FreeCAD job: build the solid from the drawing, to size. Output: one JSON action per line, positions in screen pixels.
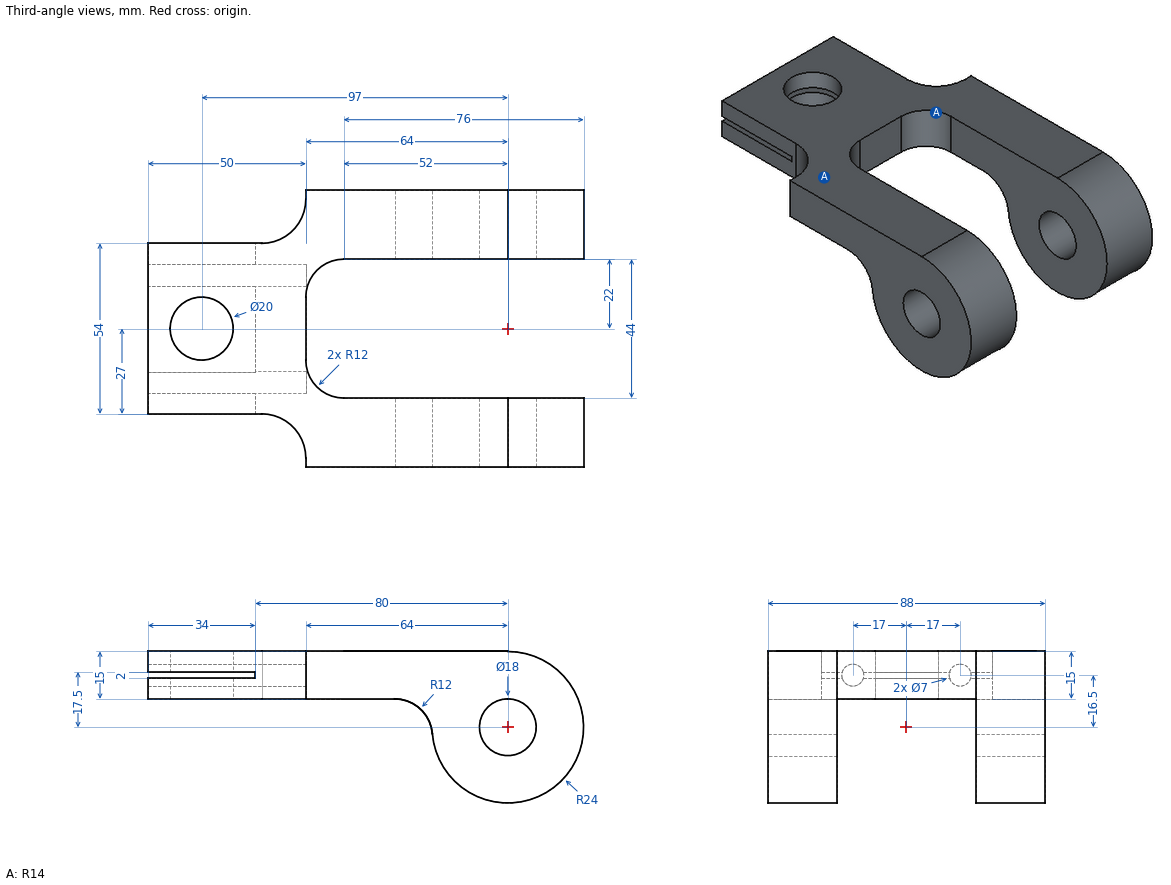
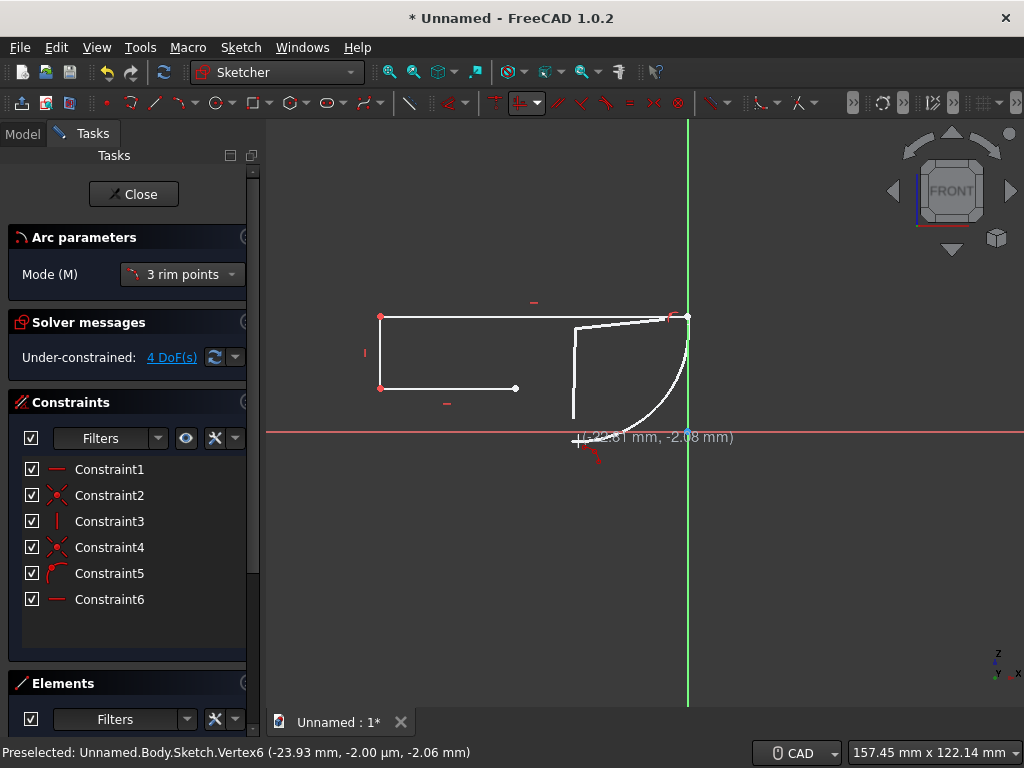
{"action": "left_click", "coordinate": [773, 510]}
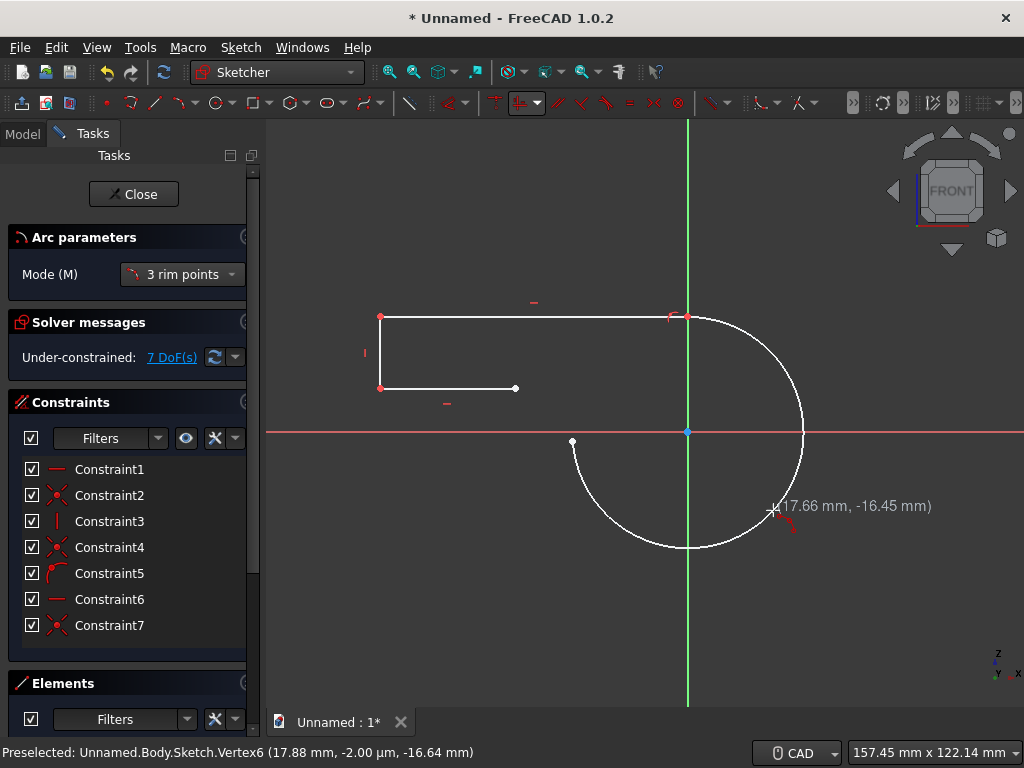
{"action": "scroll", "coordinate": [573, 441], "scroll_direction": "up", "scroll_amount": 3}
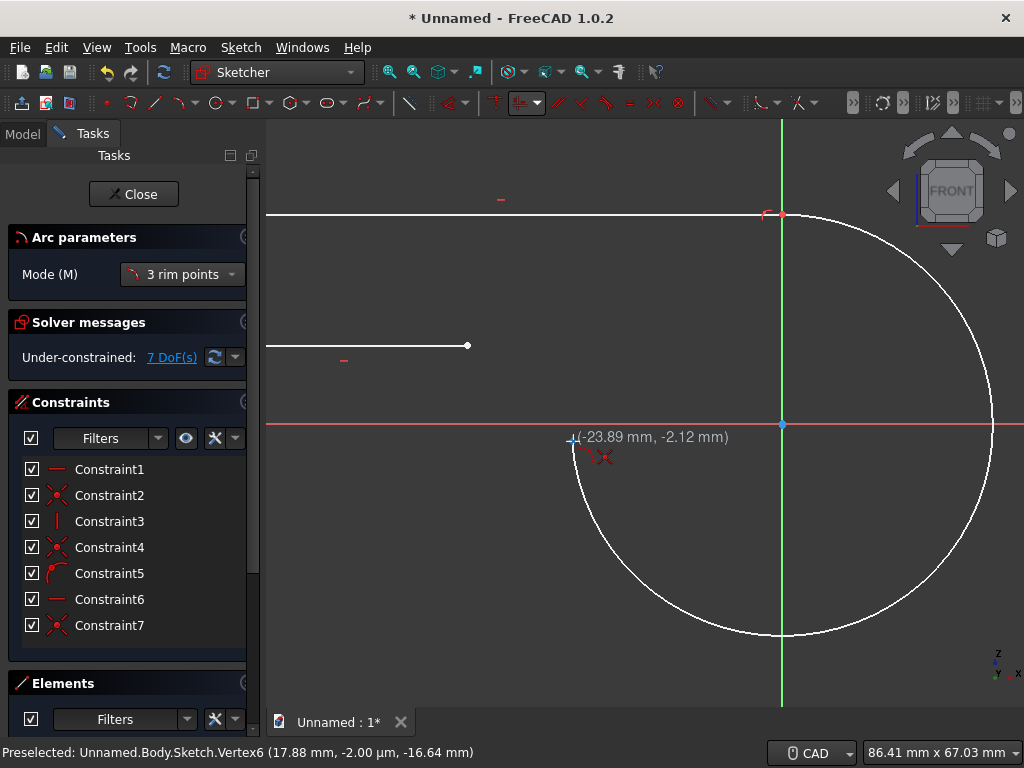
{"action": "left_click", "coordinate": [572, 442]}
{"action": "left_click", "coordinate": [467, 346]}
{"action": "left_click", "coordinate": [539, 373]}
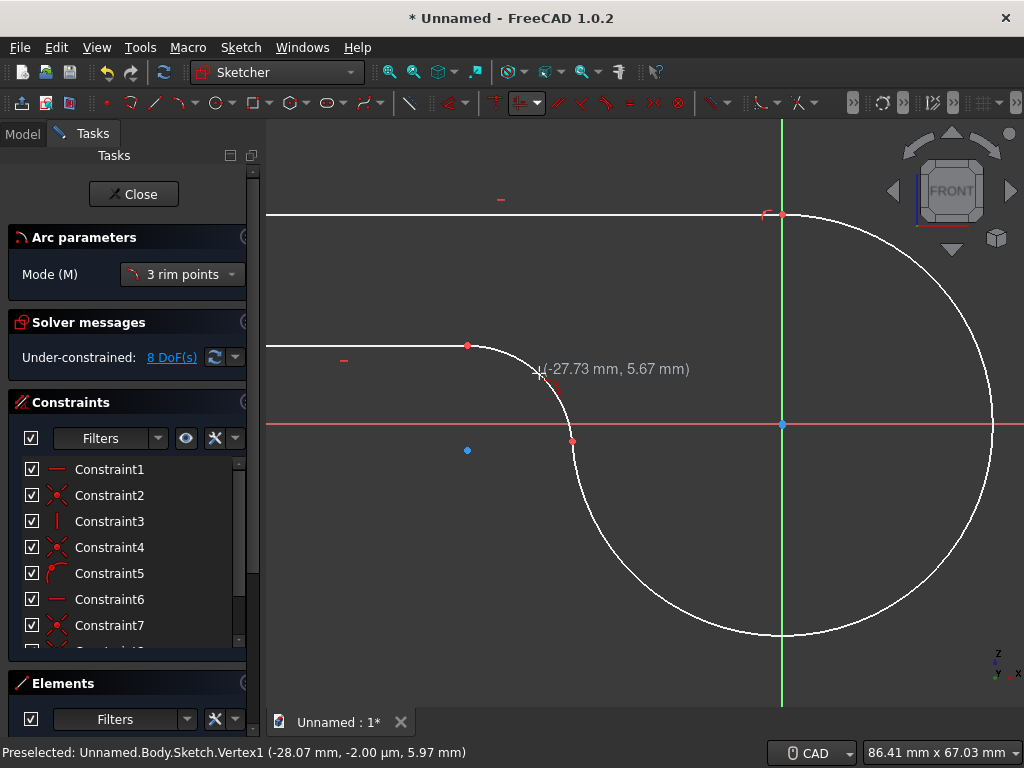
{"action": "left_click", "coordinate": [216, 104]}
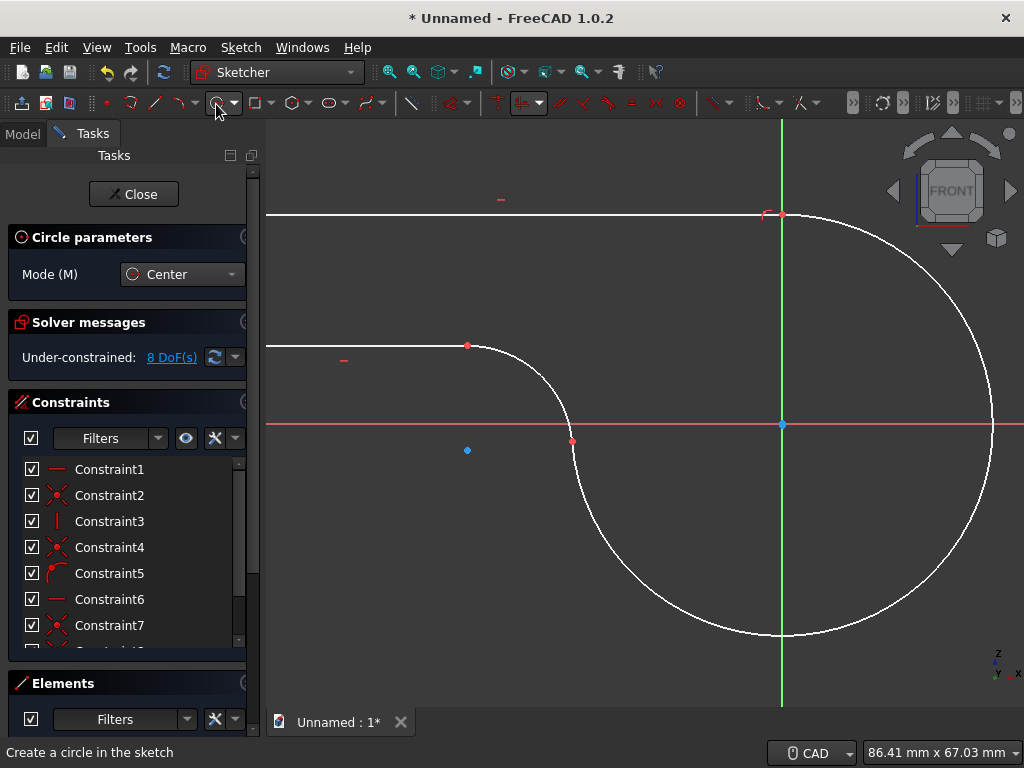
{"action": "left_click", "coordinate": [782, 424]}
{"action": "left_click", "coordinate": [838, 368]}
{"action": "key", "text": "Escape"}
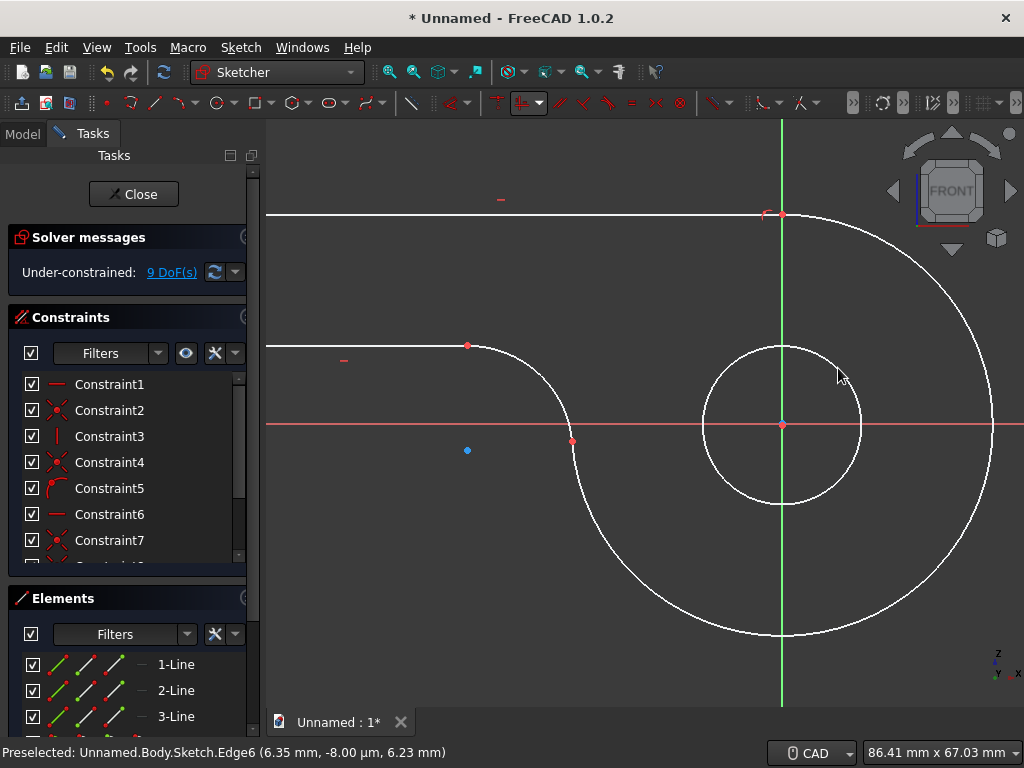
{"action": "left_click", "coordinate": [393, 346]}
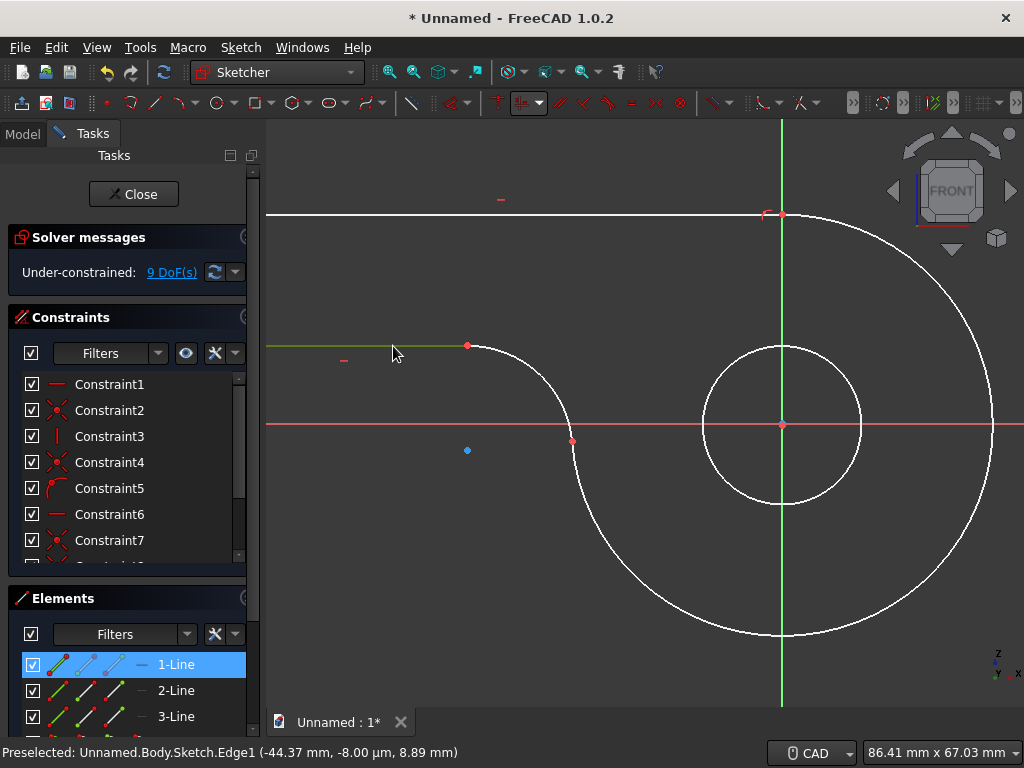
{"action": "left_click", "coordinate": [558, 398]}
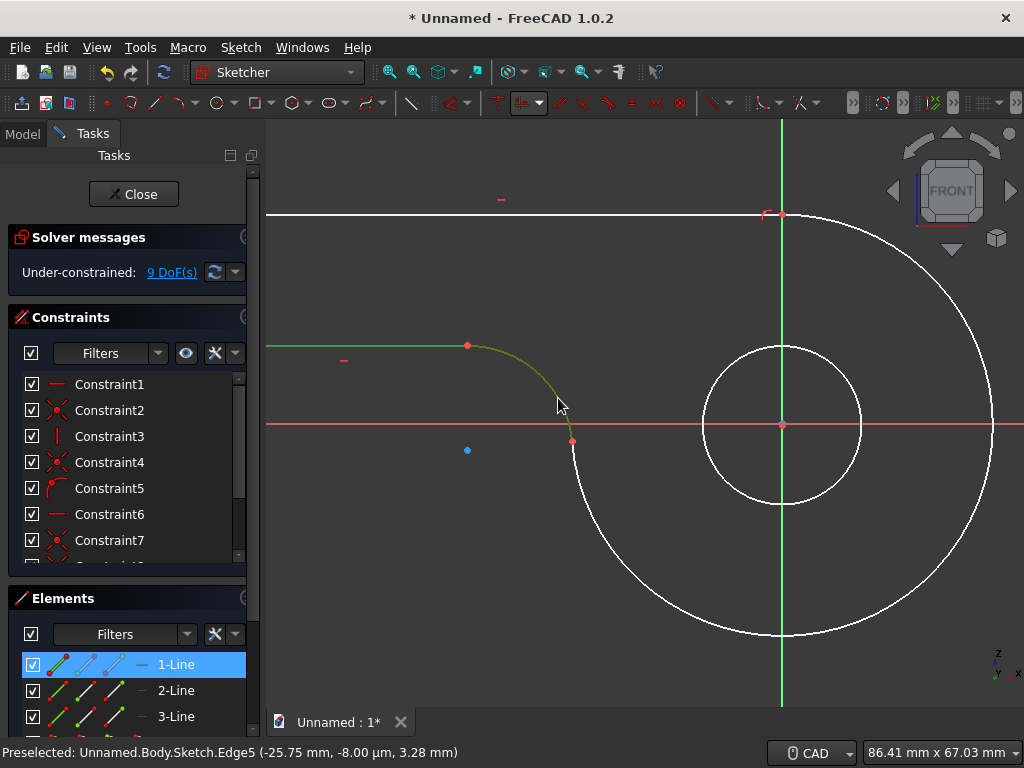
{"action": "left_click", "coordinate": [608, 104]}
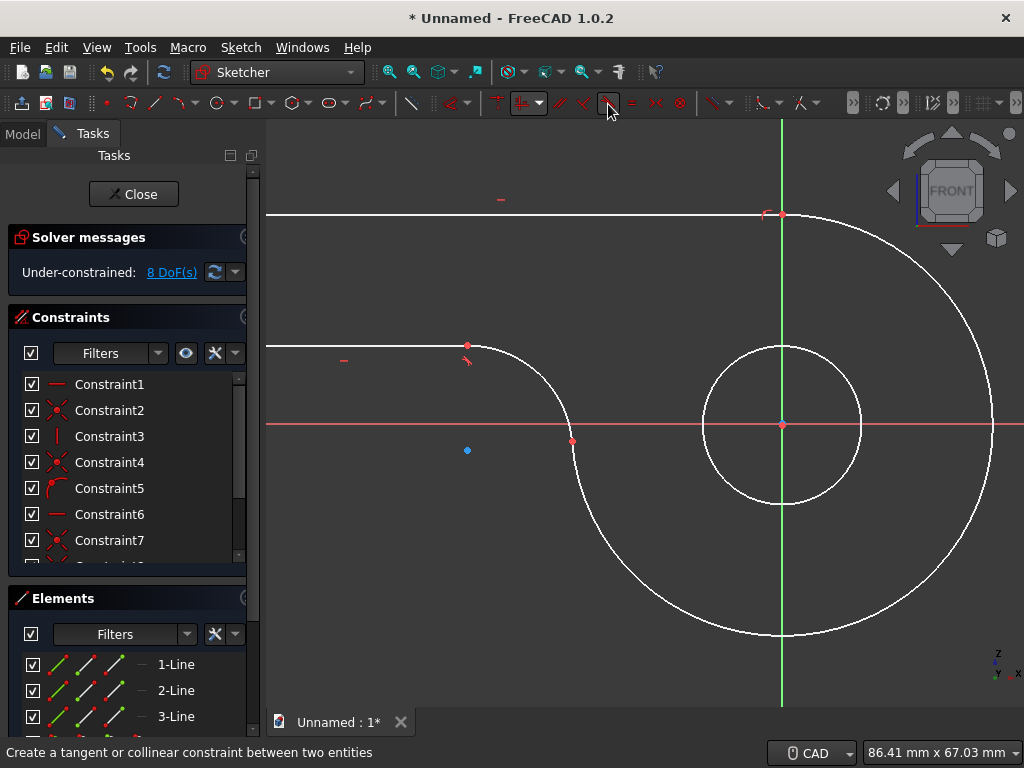
{"action": "left_click", "coordinate": [389, 215]}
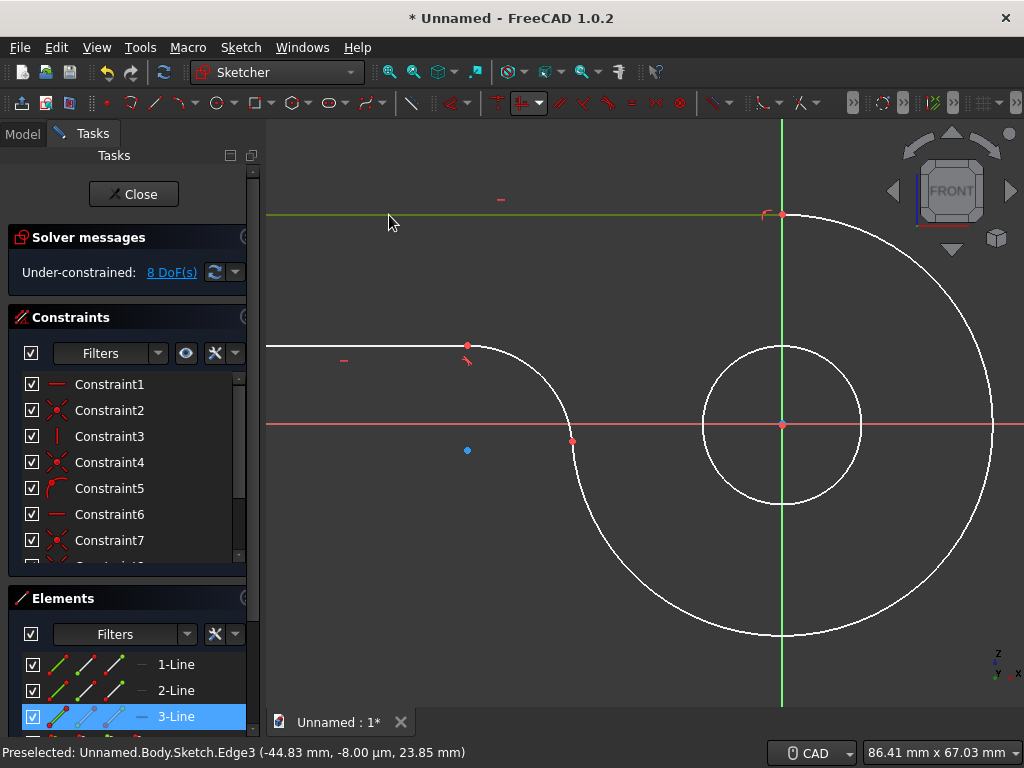
{"action": "left_click", "coordinate": [761, 635]}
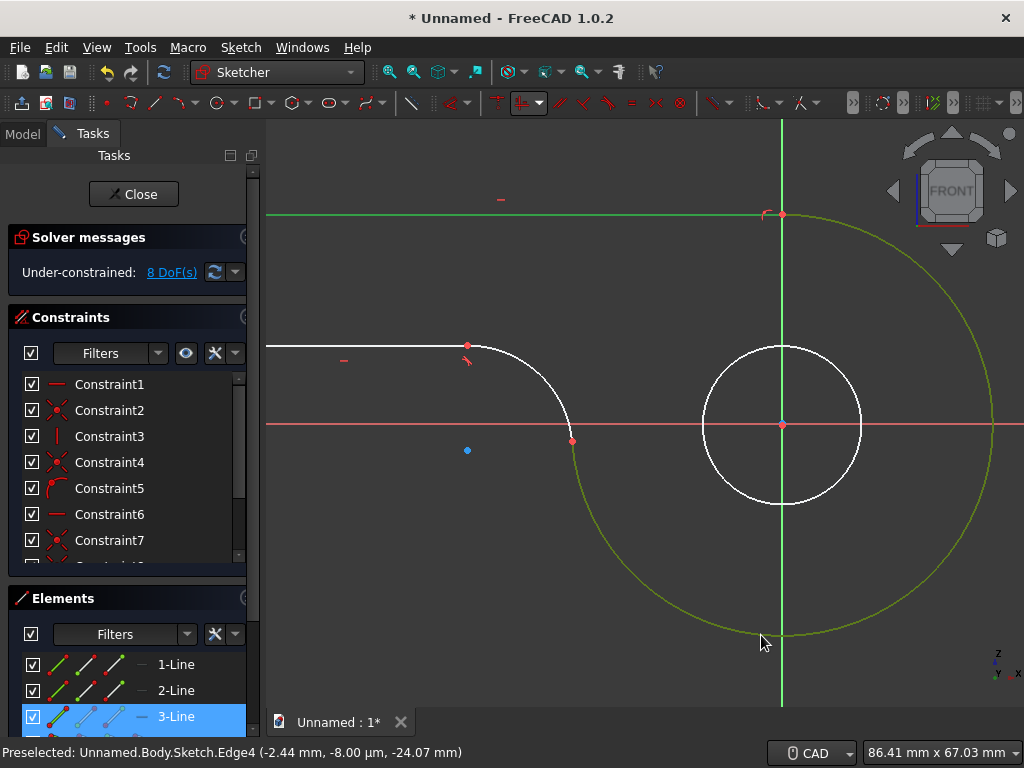
{"action": "left_click", "coordinate": [608, 104]}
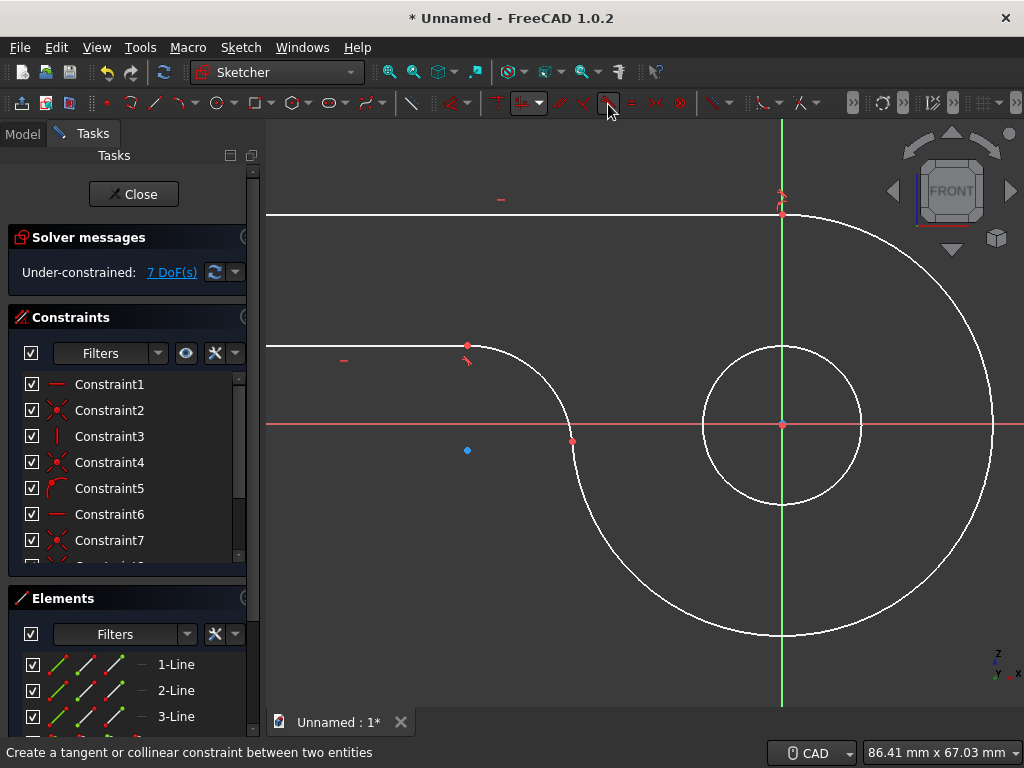
{"action": "left_click", "coordinate": [761, 635]}